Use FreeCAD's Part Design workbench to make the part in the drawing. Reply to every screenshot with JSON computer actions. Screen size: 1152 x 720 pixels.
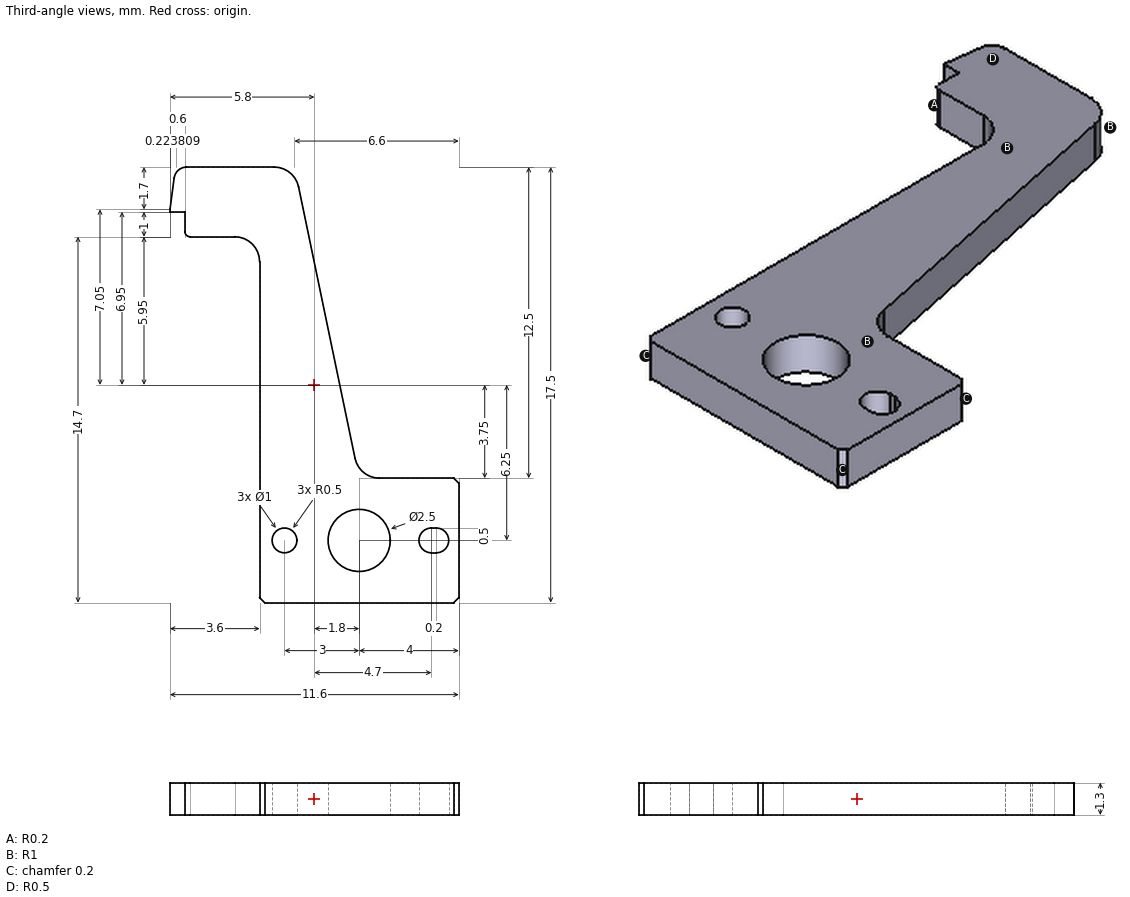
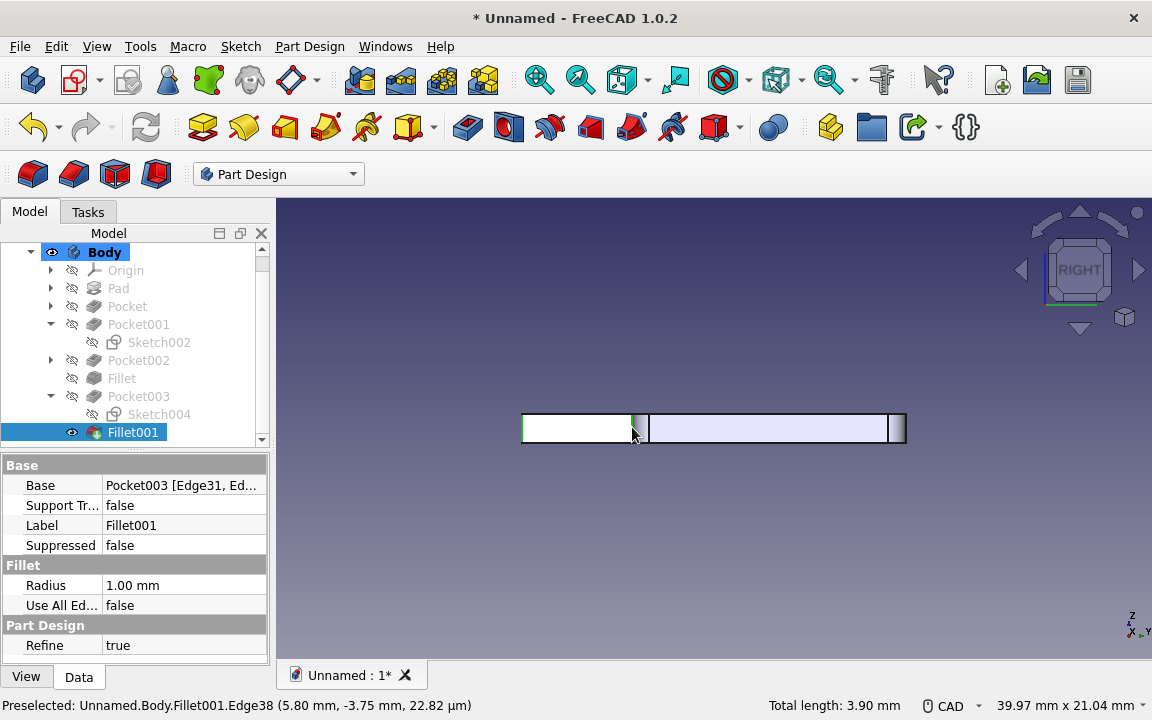
{"action": "left_click", "coordinate": [74, 174]}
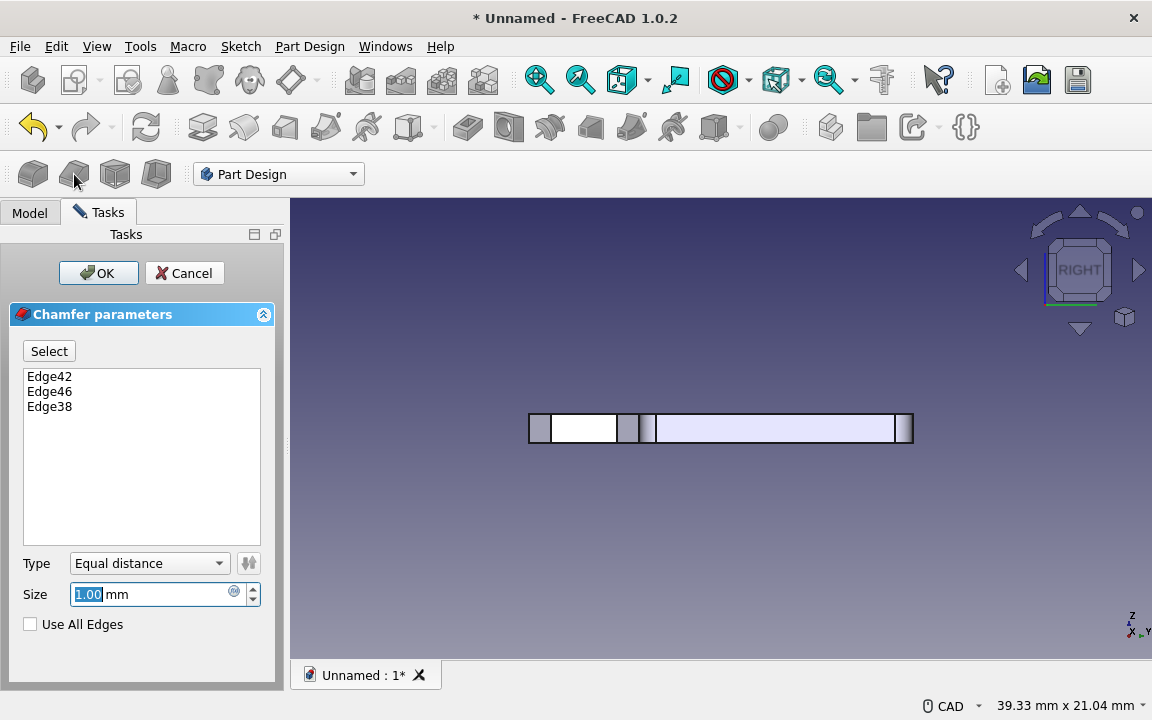
{"action": "type", "text": "0.2"}
{"action": "key", "text": "Tab"}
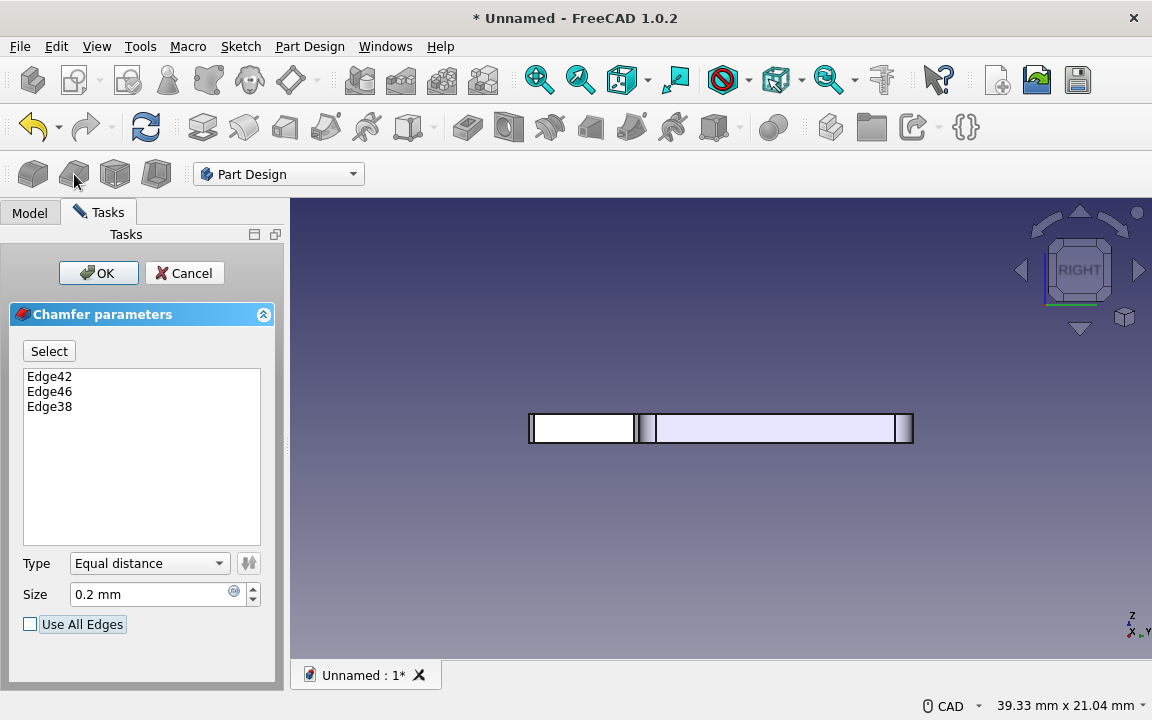
{"action": "left_click", "coordinate": [99, 273]}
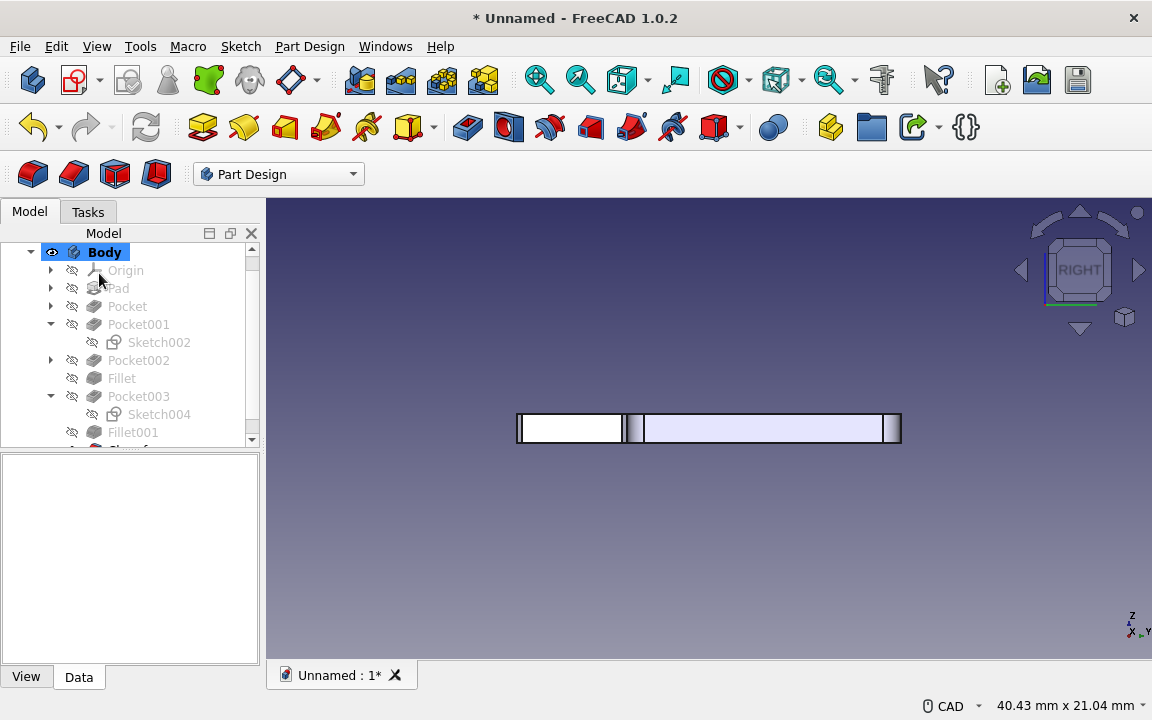
{"action": "key", "text": "v f"}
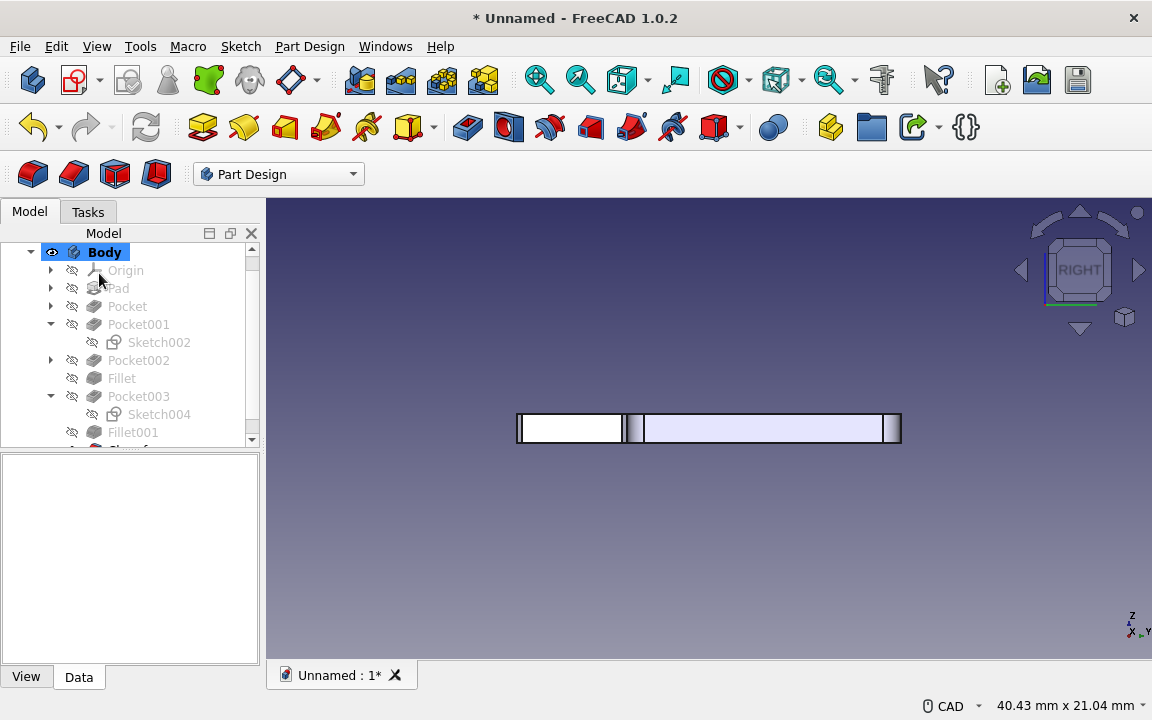
{"action": "key", "text": "0"}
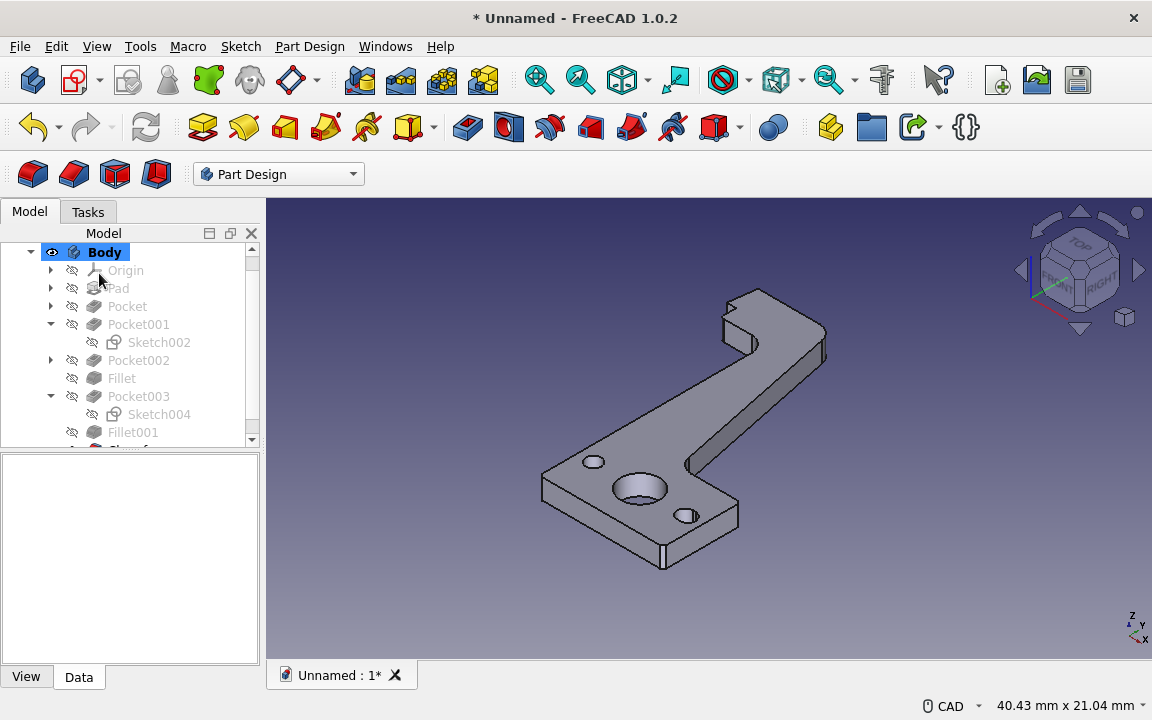
{"action": "key", "text": "2"}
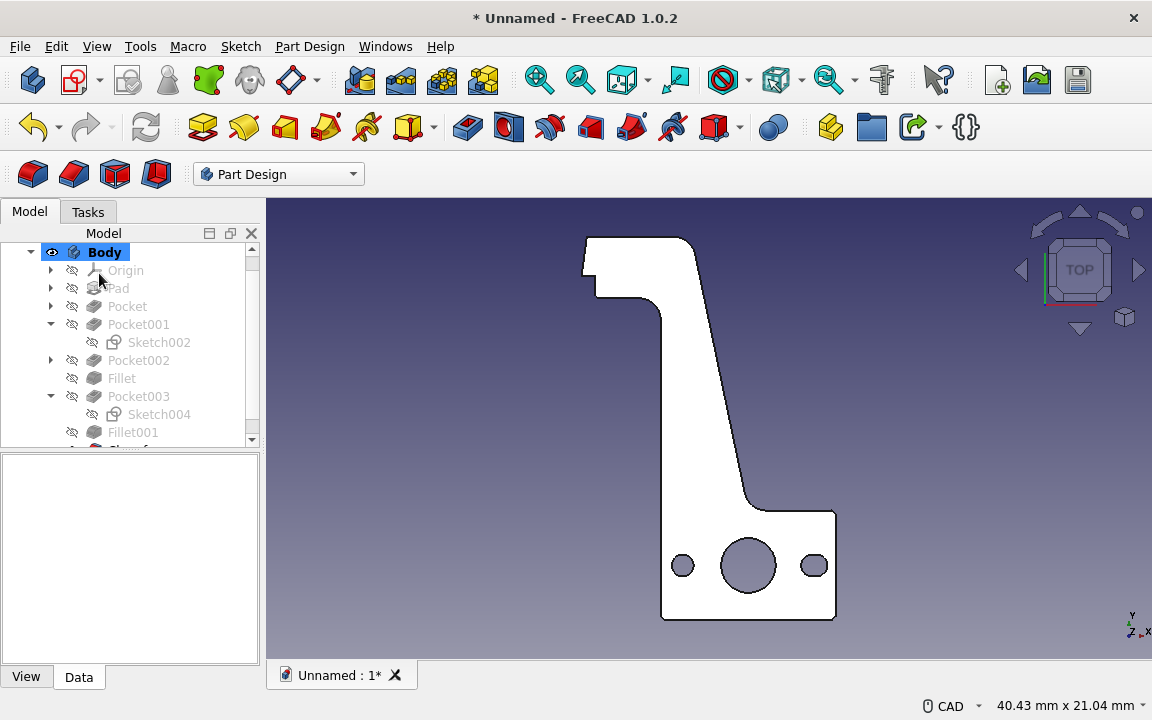
{"action": "key", "text": "1"}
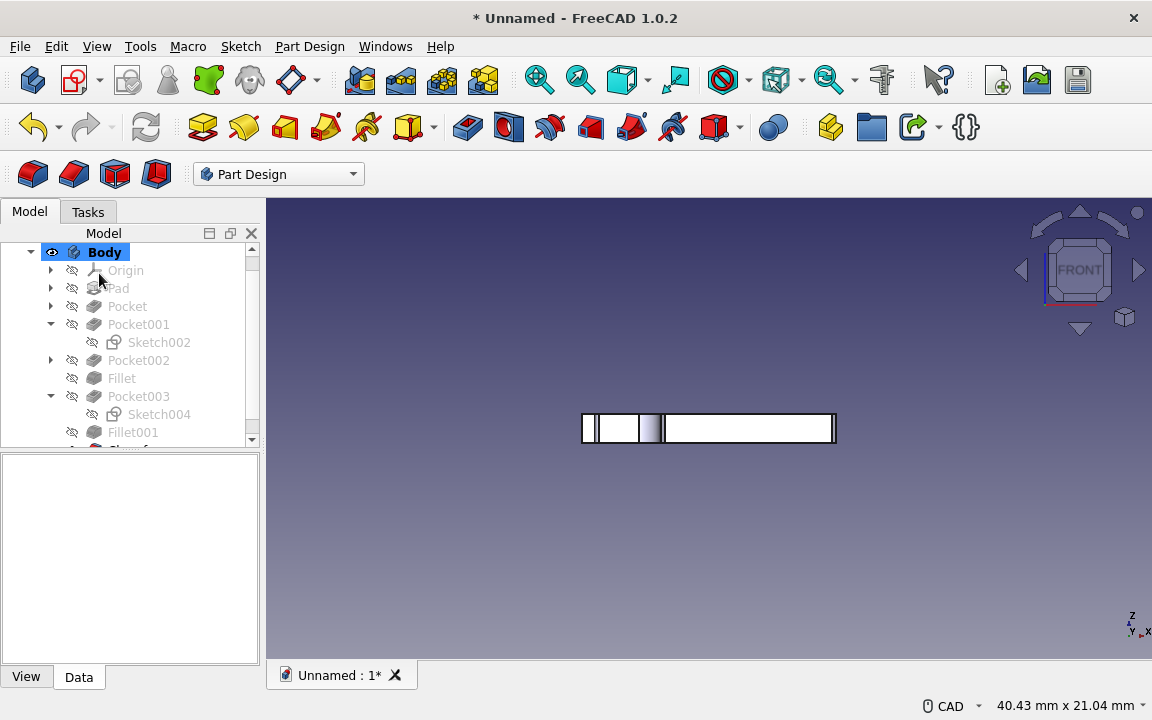
{"action": "key", "text": "v f"}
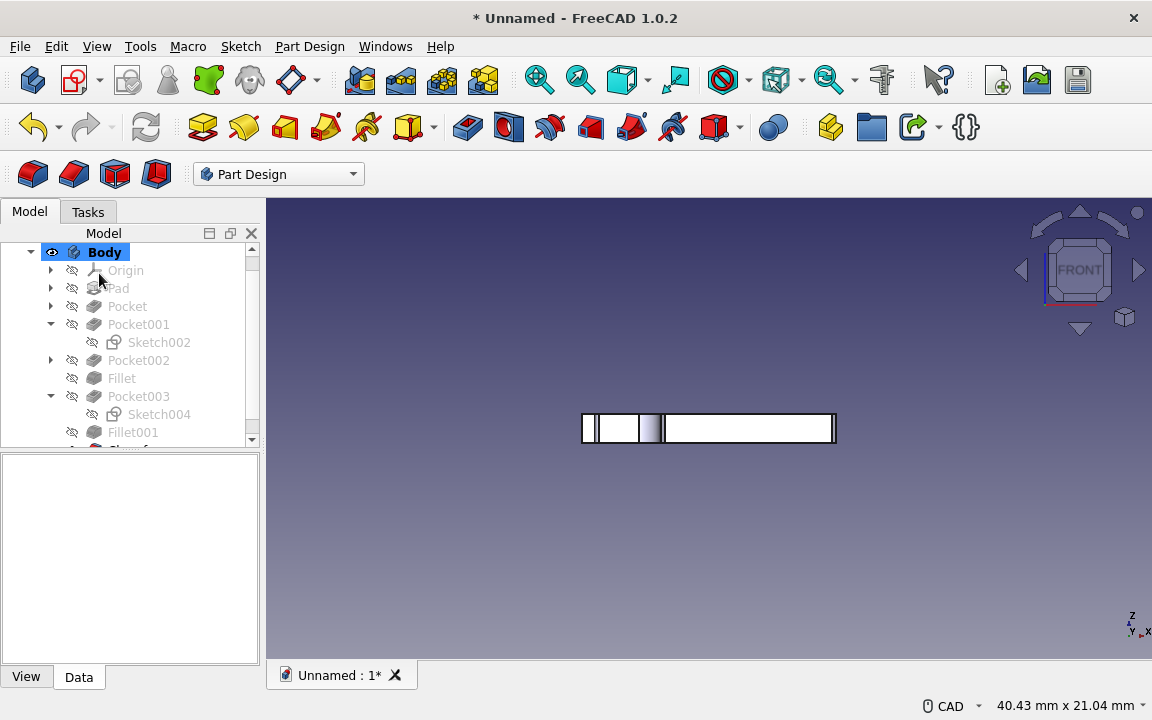
{"action": "key", "text": "3"}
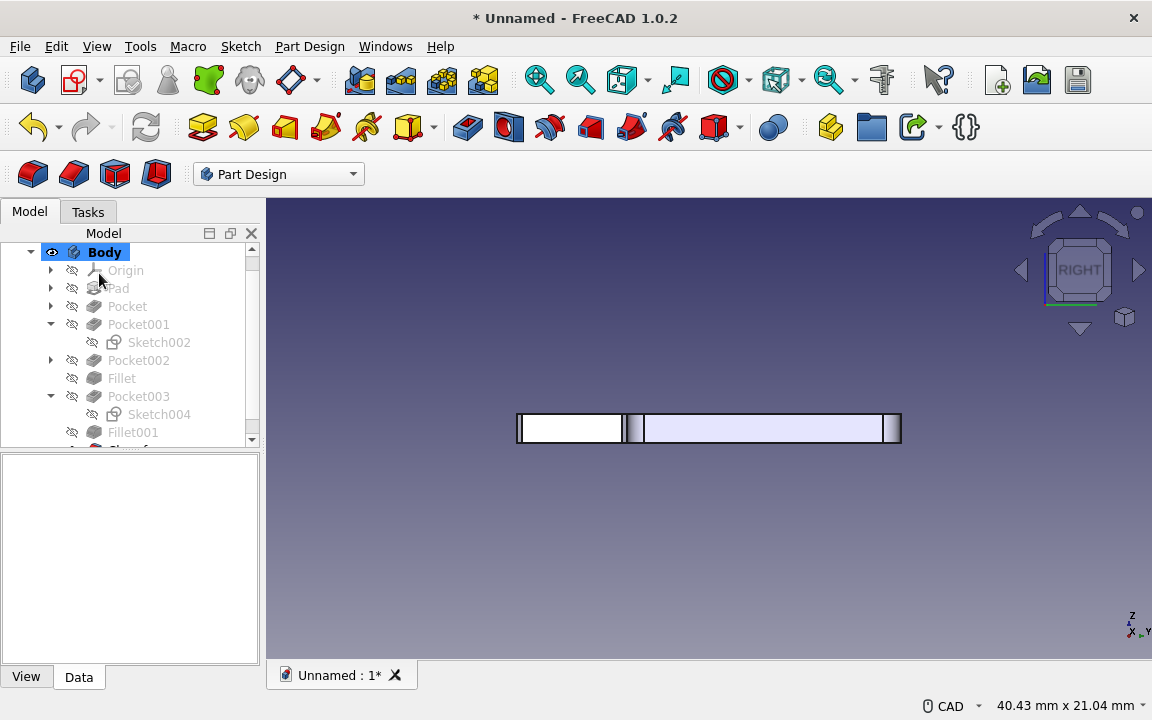
{"action": "key", "text": "v f"}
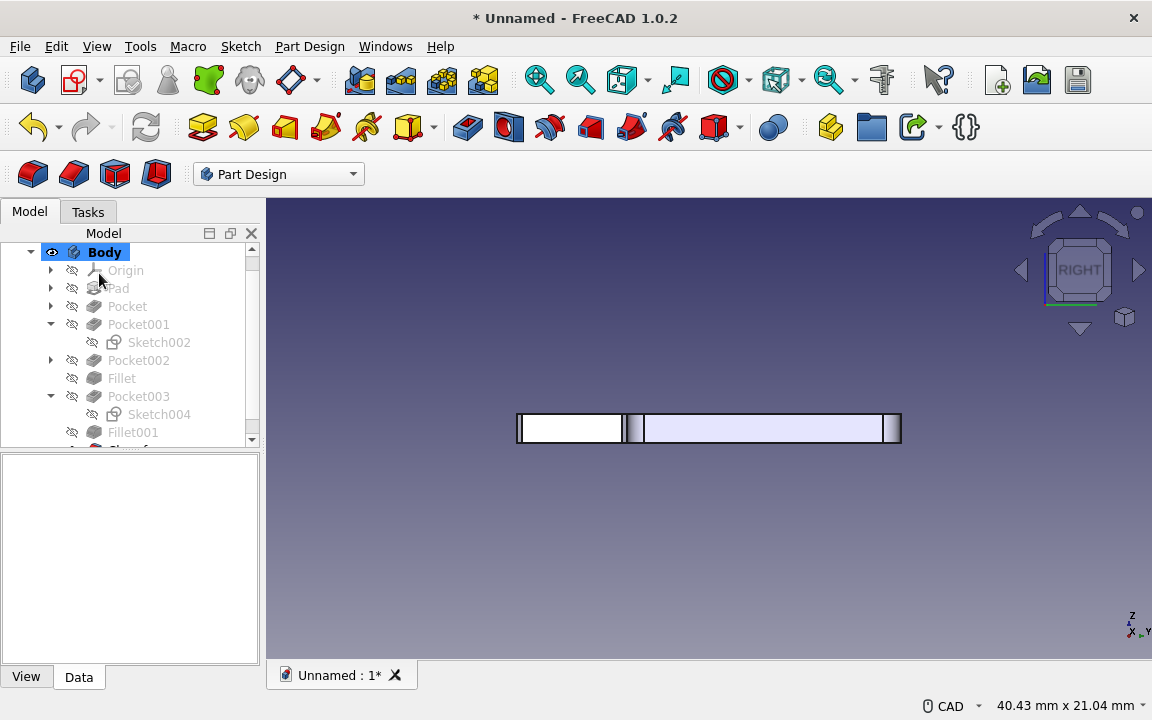
{"action": "key", "text": "5"}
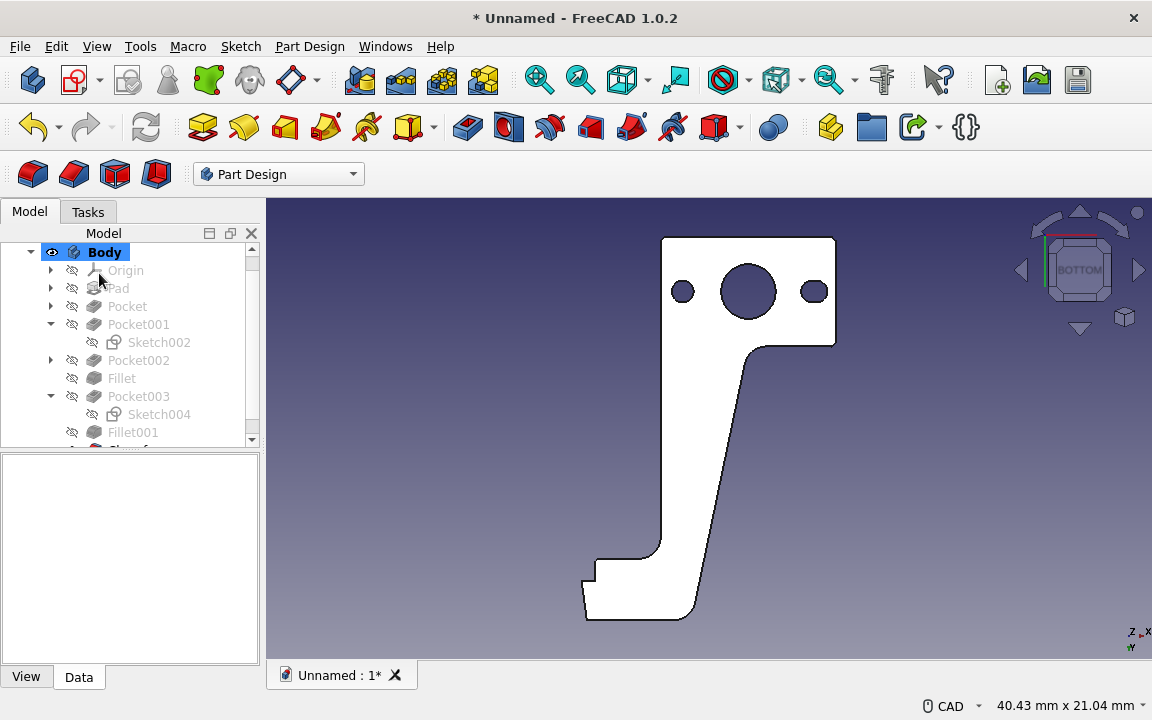
{"action": "key", "text": "4"}